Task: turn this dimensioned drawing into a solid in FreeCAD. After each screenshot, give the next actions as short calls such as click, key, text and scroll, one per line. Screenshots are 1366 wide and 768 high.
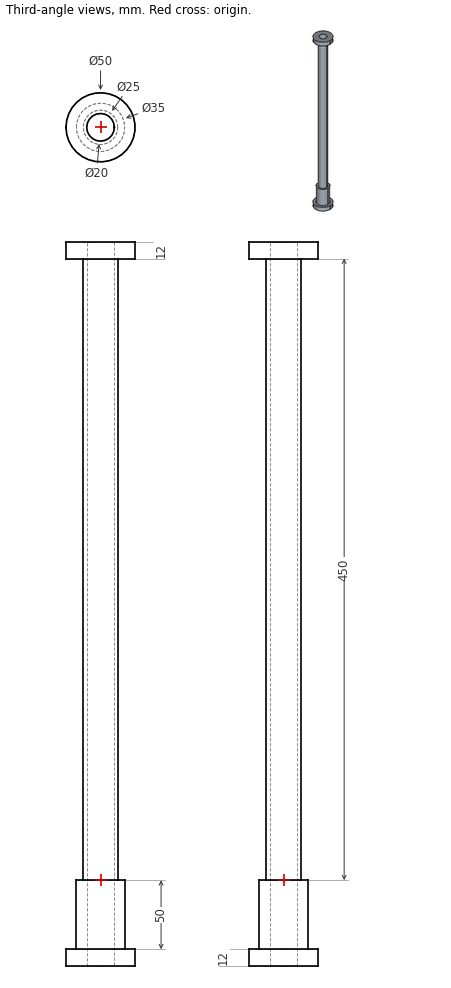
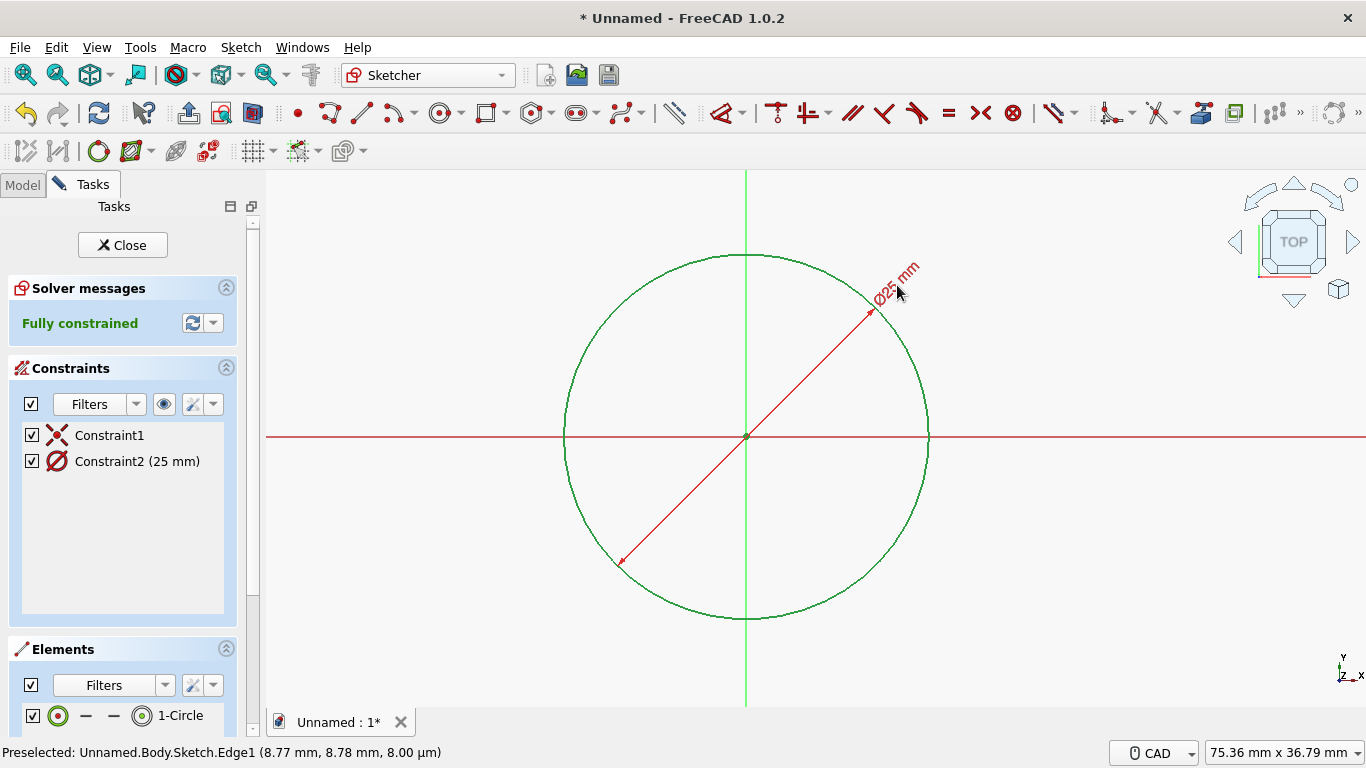
click(123, 245)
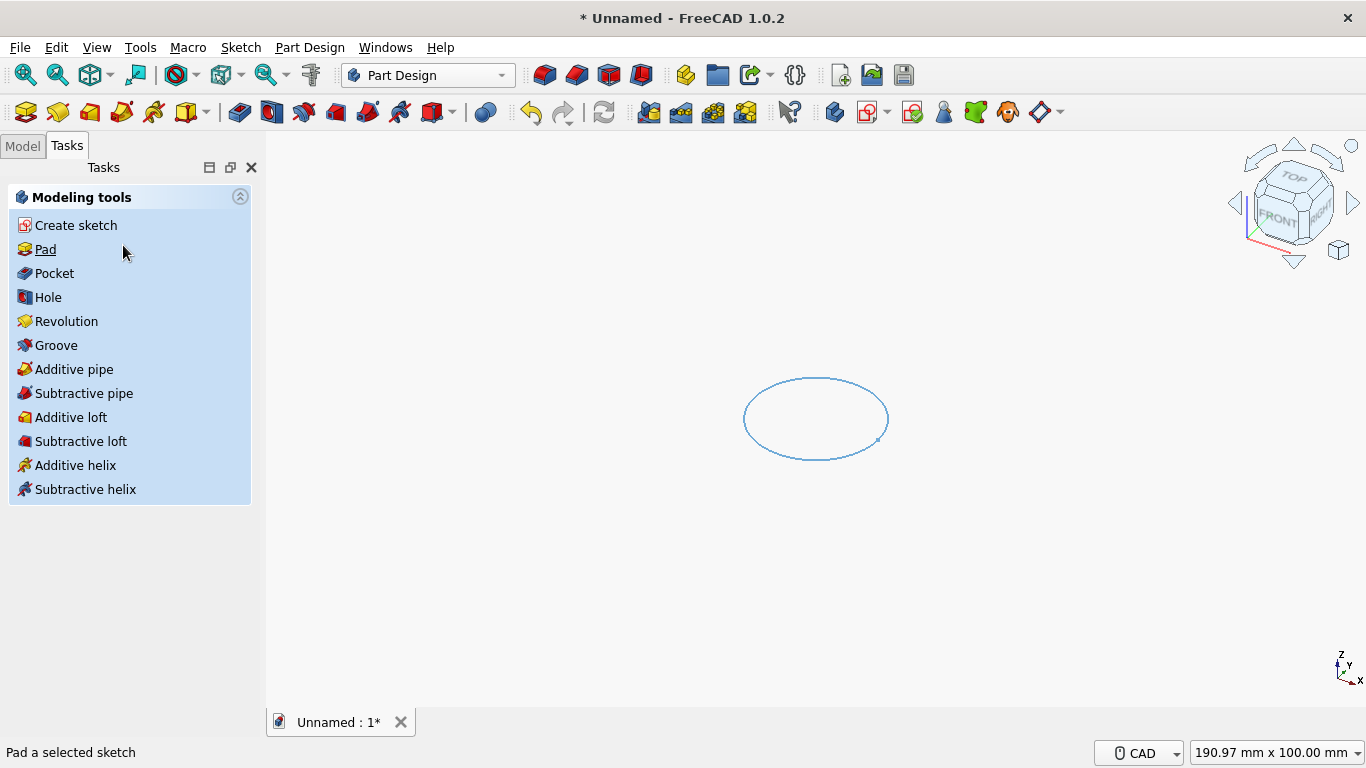
click(26, 112)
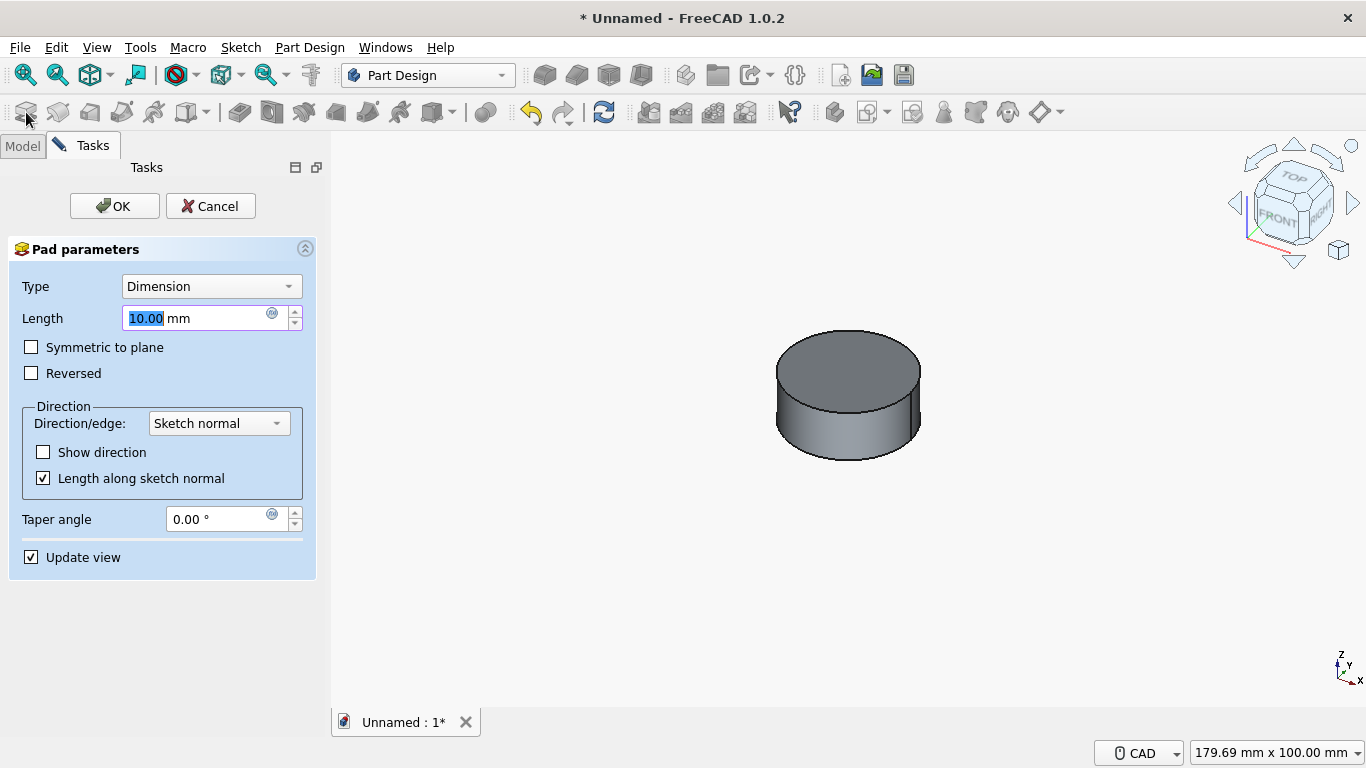
text(450)
key(Tab)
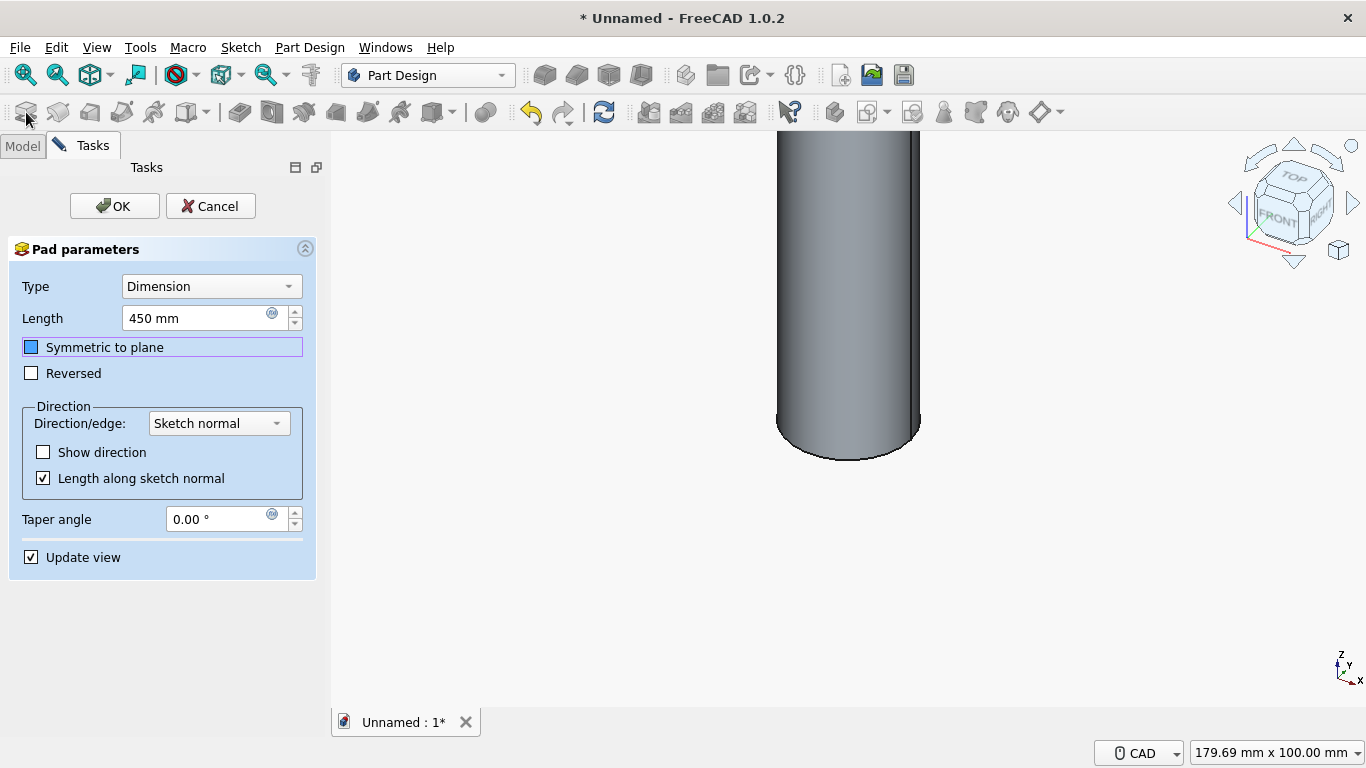
click(115, 206)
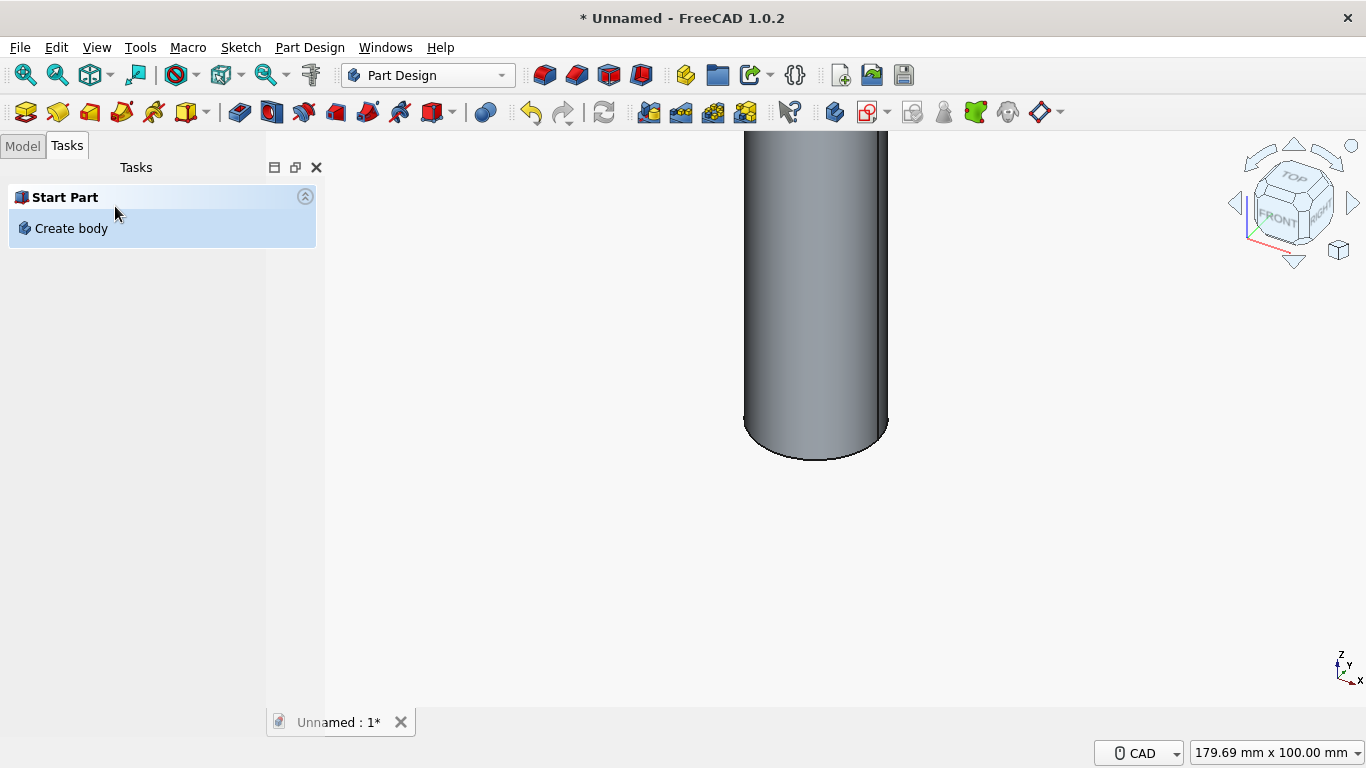
click(26, 76)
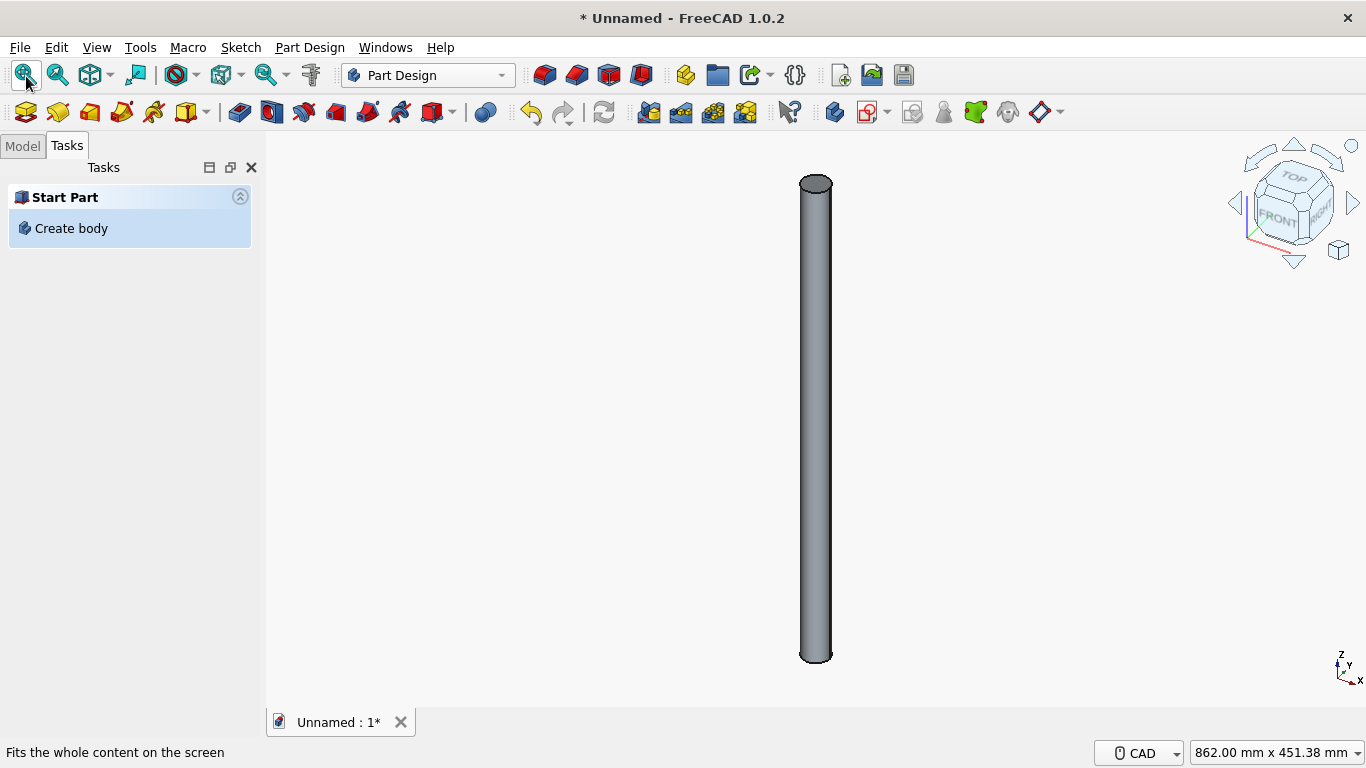
click(868, 112)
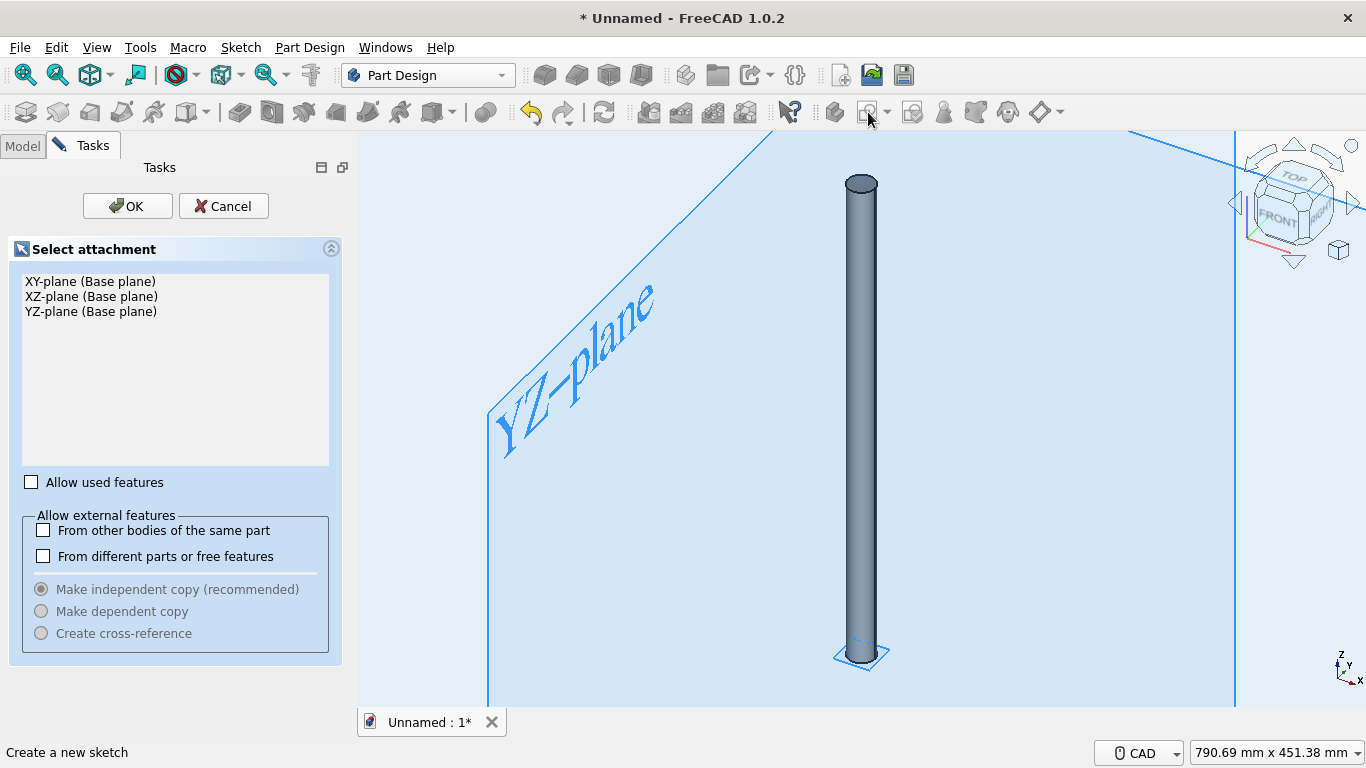
click(82, 282)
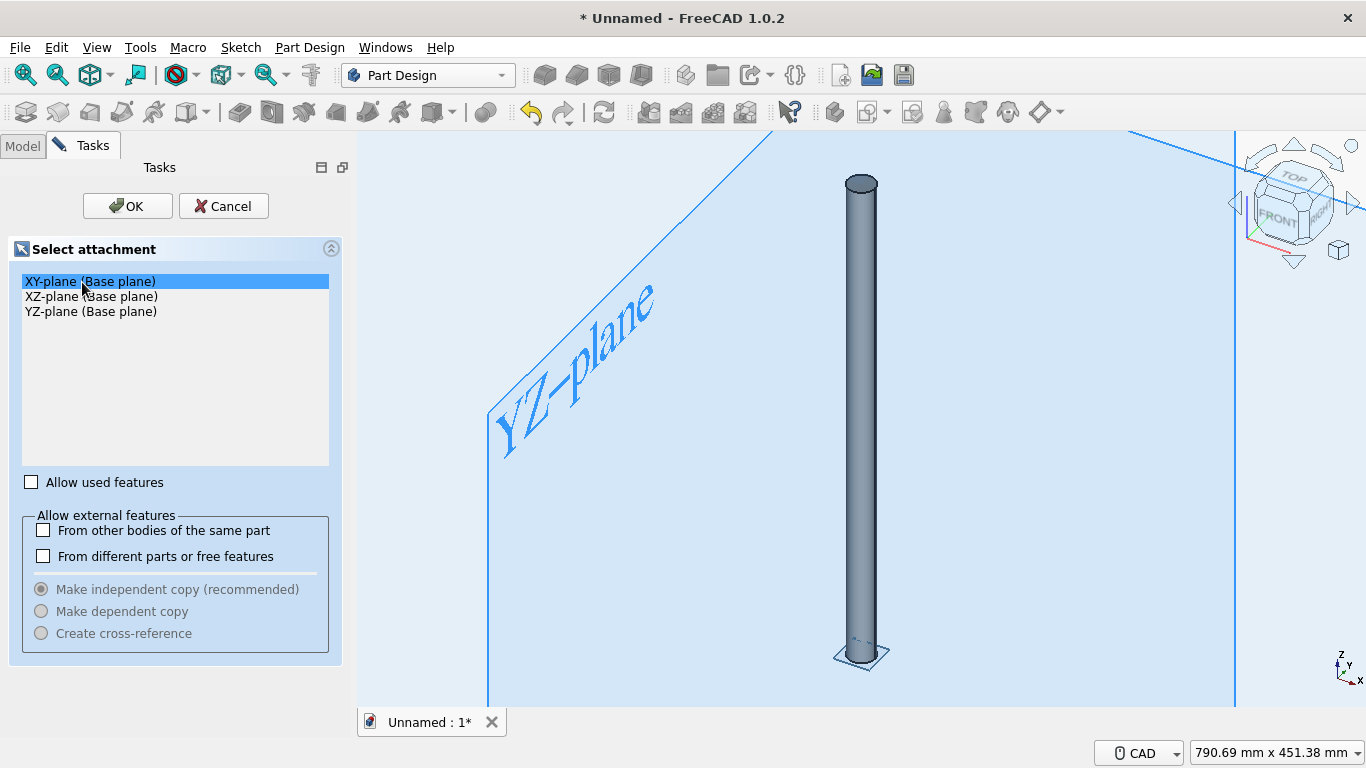
click(128, 206)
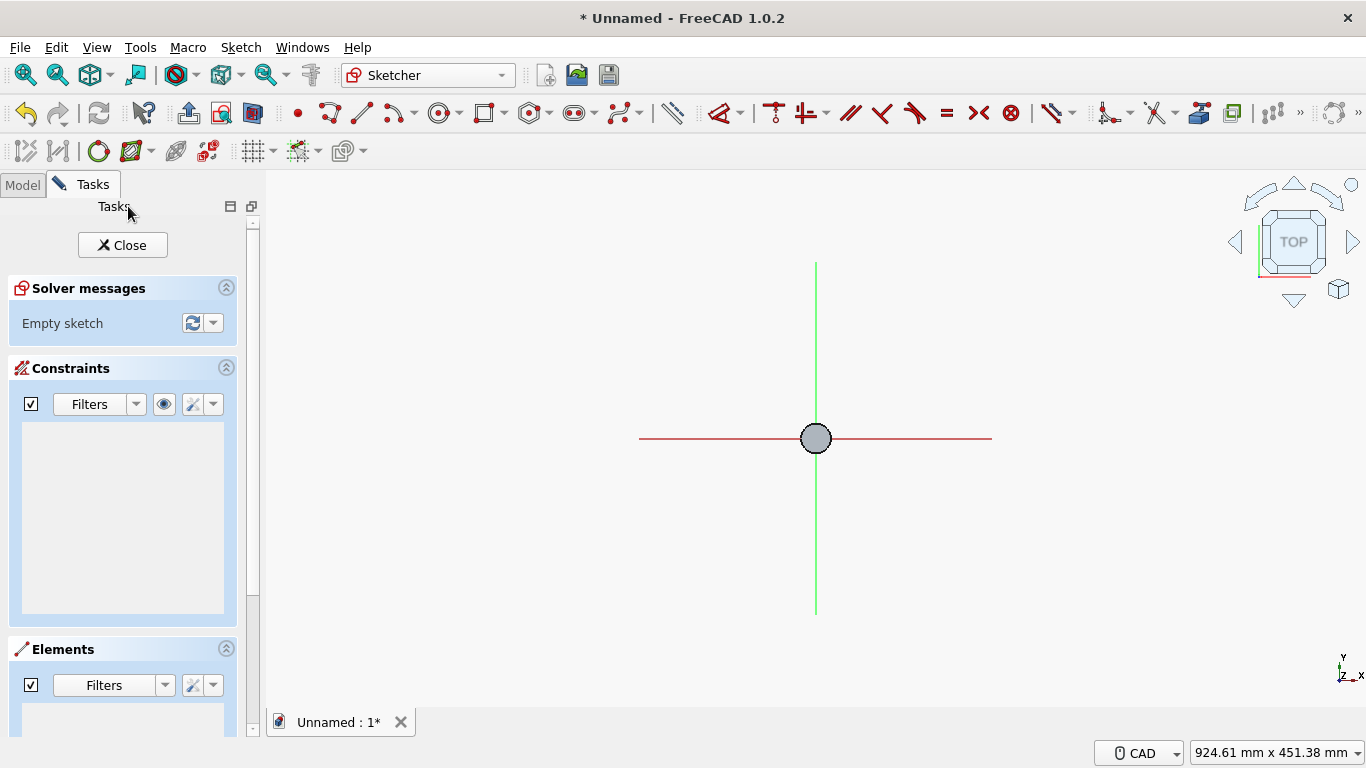
click(254, 114)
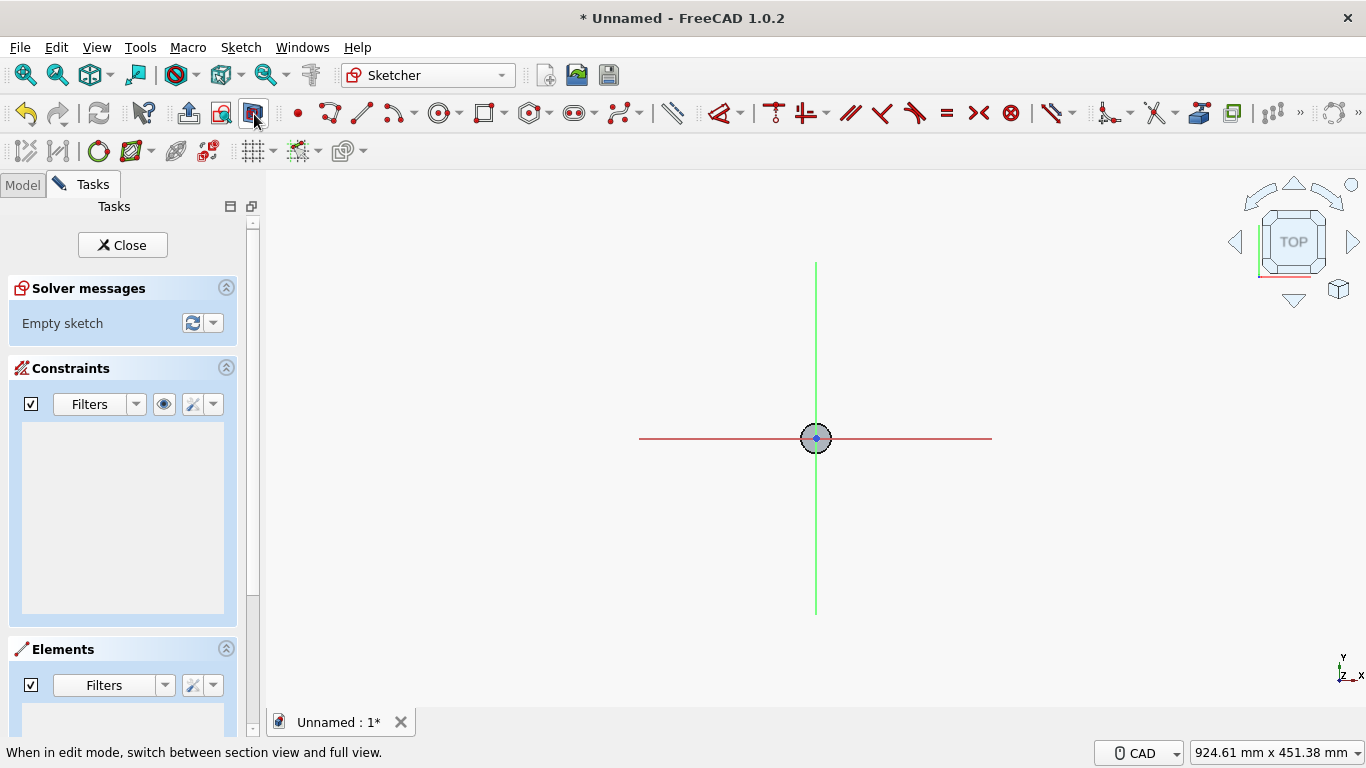
scroll(827, 438, up, 10)